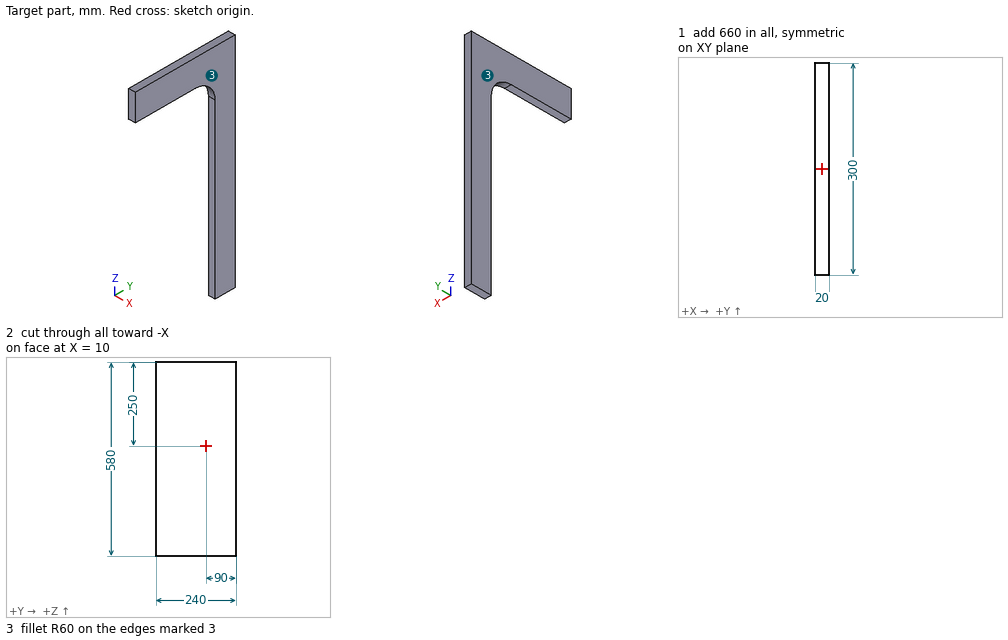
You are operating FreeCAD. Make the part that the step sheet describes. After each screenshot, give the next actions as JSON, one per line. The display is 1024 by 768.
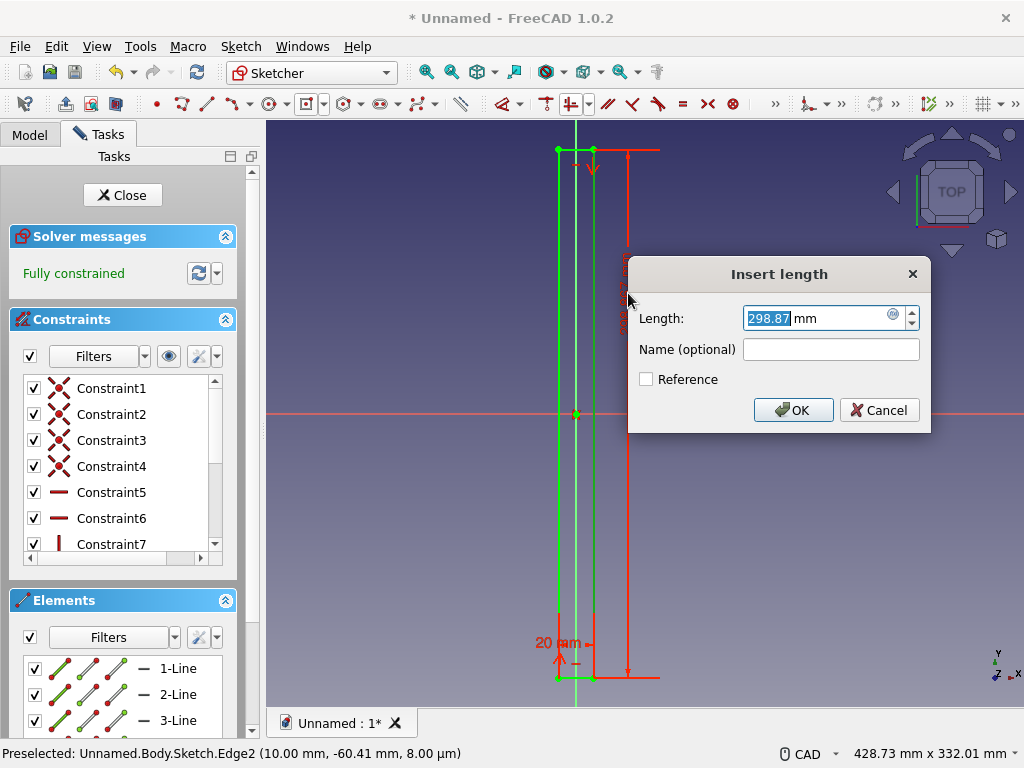
{"action": "type", "text": "300"}
{"action": "key", "text": "Return"}
{"action": "key", "text": "Escape"}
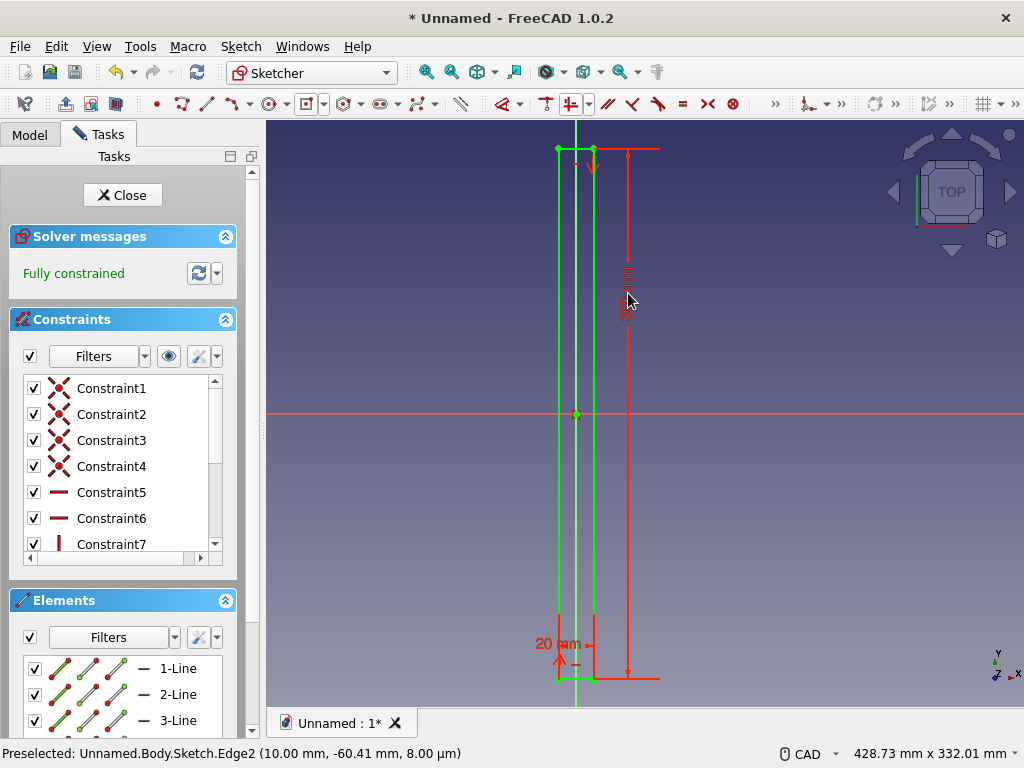
{"action": "left_click", "coordinate": [123, 195]}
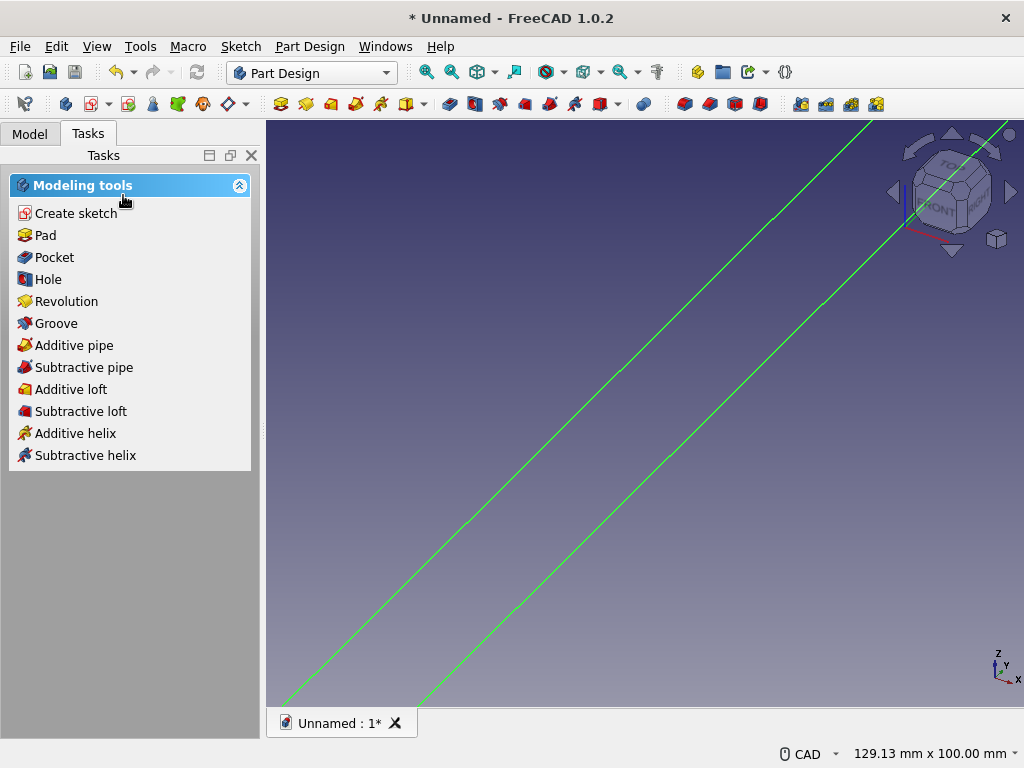
{"action": "left_click", "coordinate": [281, 104]}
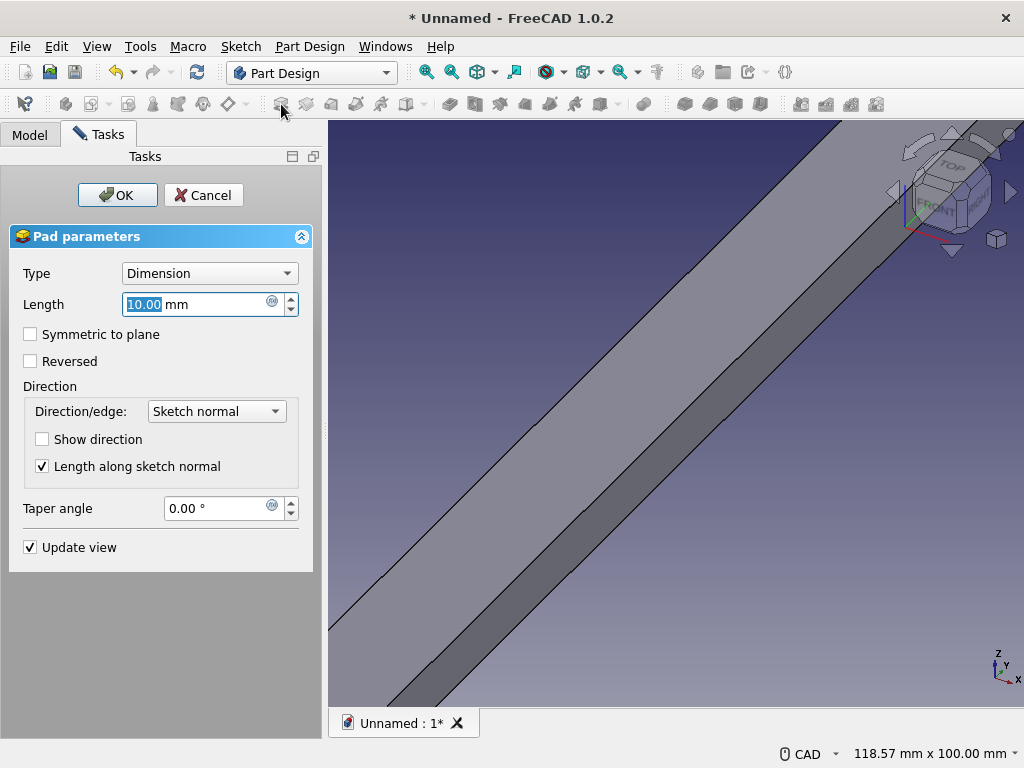
{"action": "type", "text": "660"}
{"action": "key", "text": "Tab"}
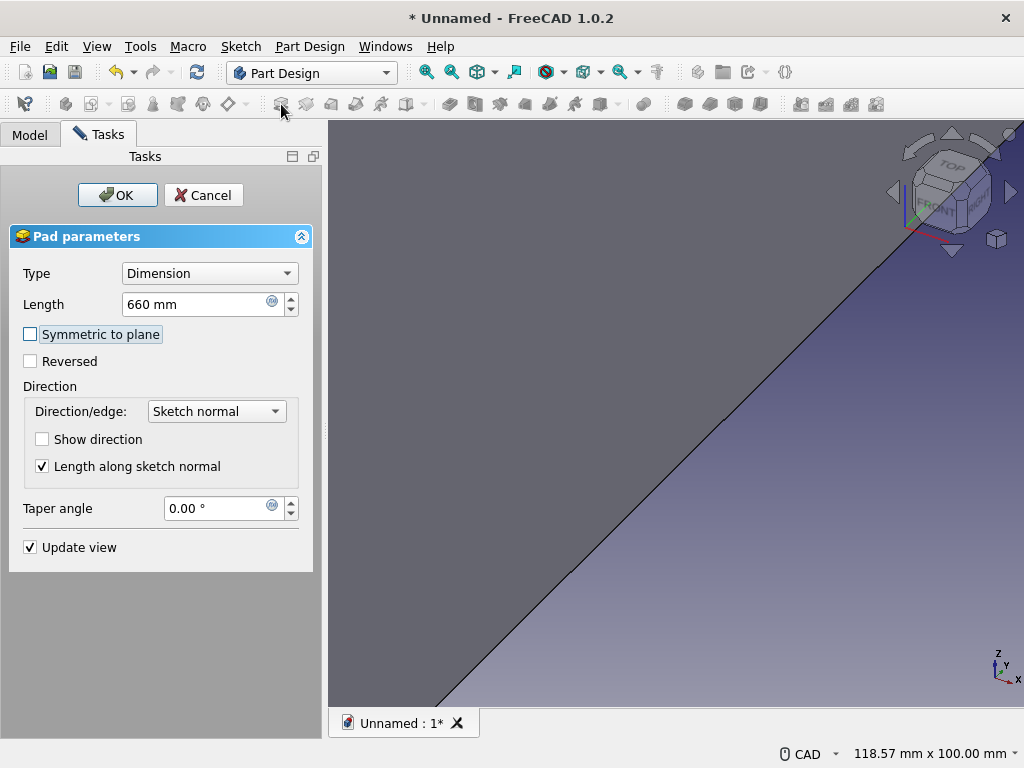
{"action": "left_click", "coordinate": [31, 334]}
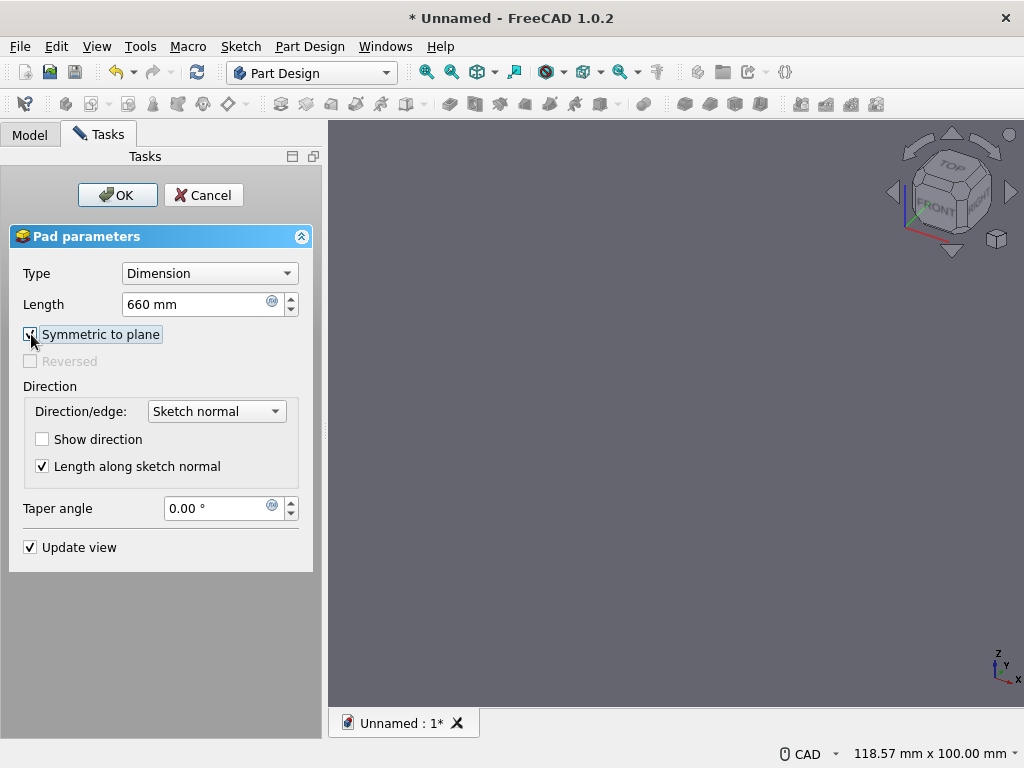
{"action": "left_click", "coordinate": [118, 195]}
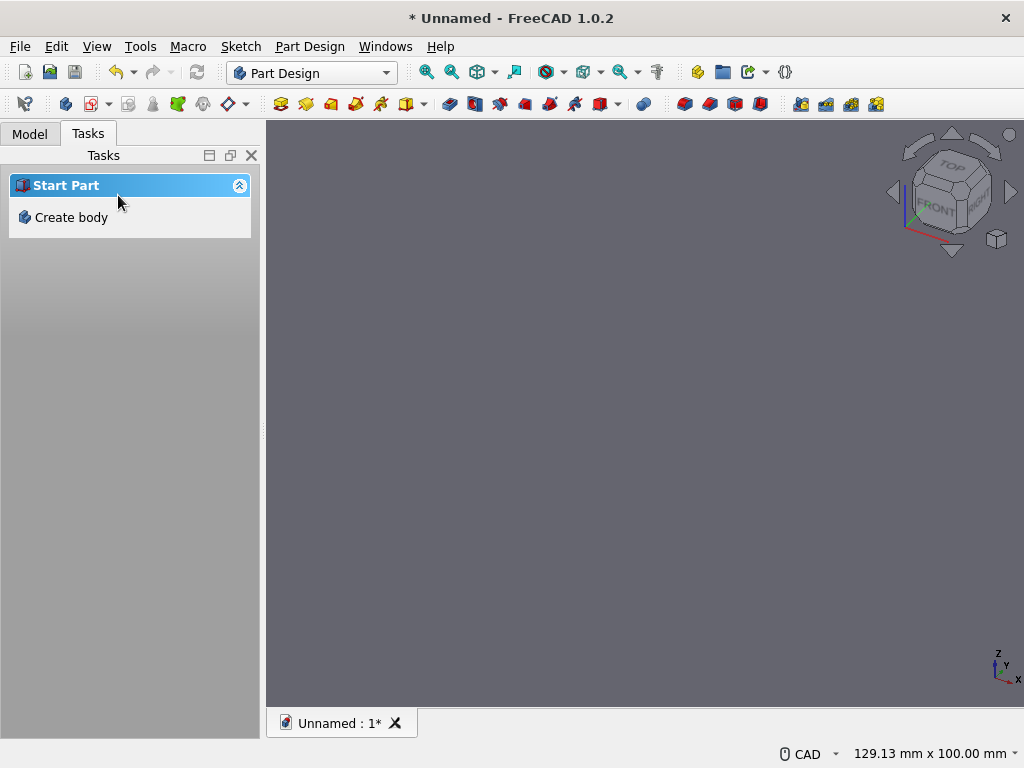
{"action": "left_click", "coordinate": [427, 72]}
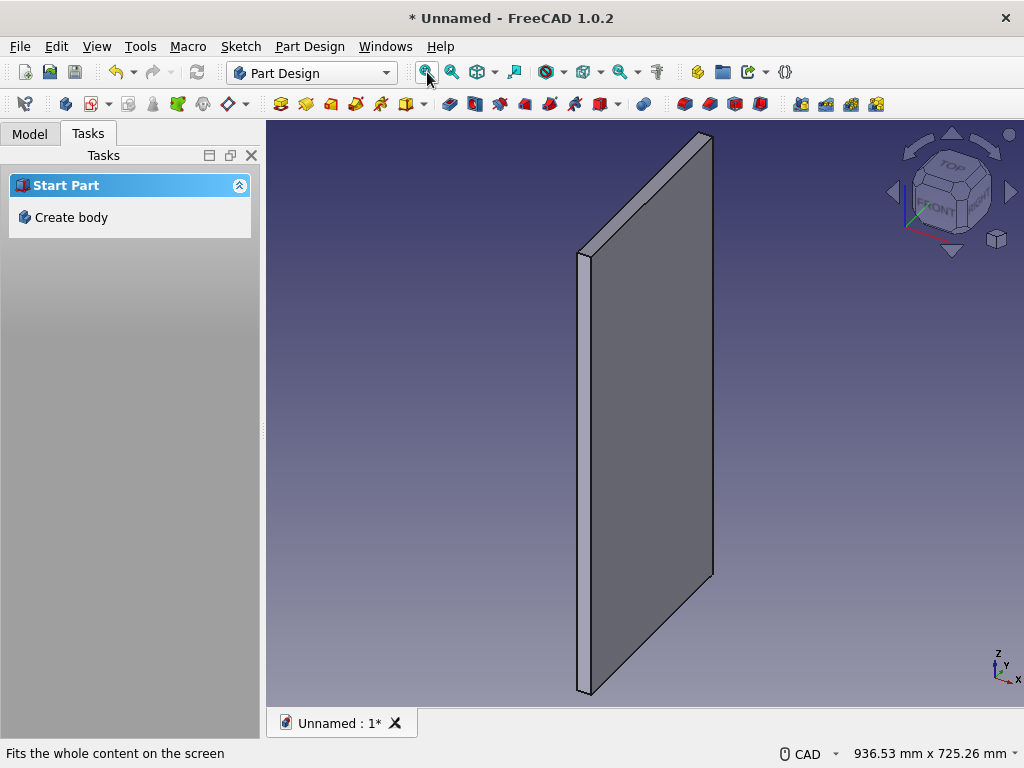
{"action": "left_click", "coordinate": [652, 352]}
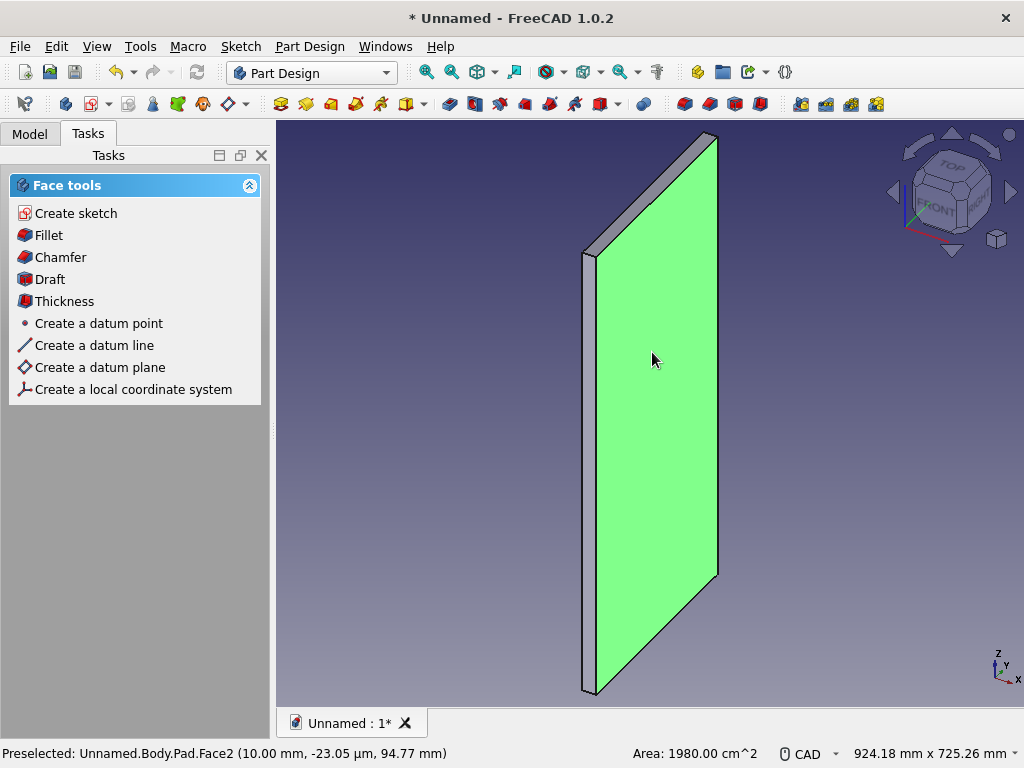
{"action": "left_click", "coordinate": [90, 104]}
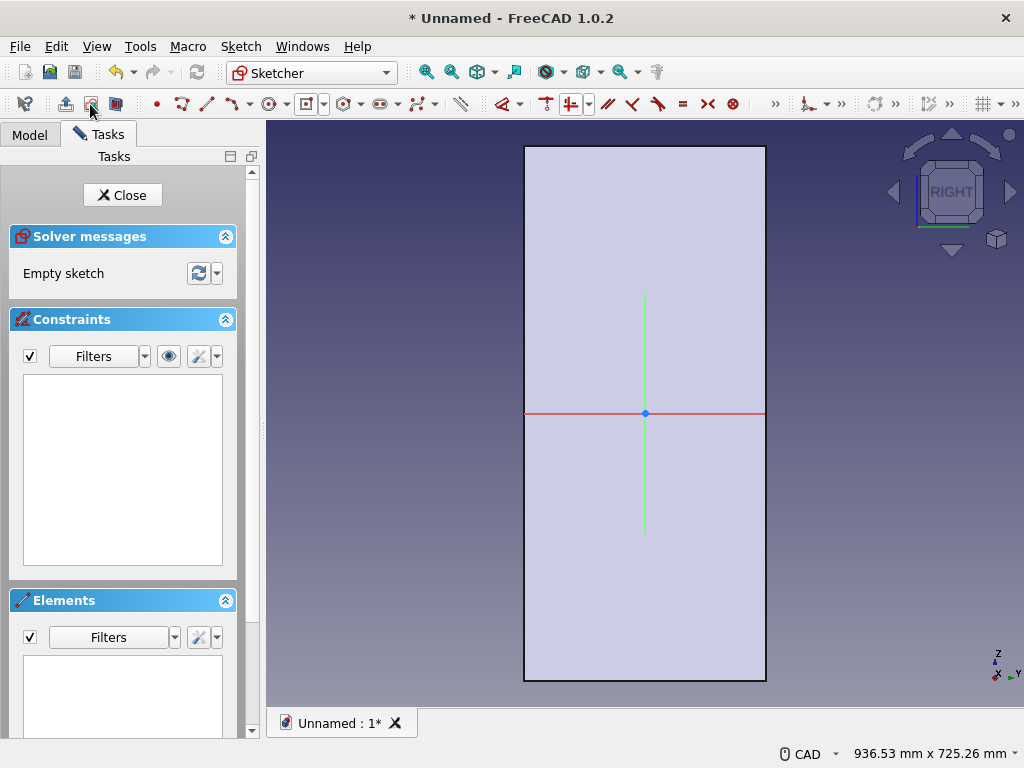
{"action": "scroll", "coordinate": [377, 267], "scroll_direction": "down", "scroll_amount": 1}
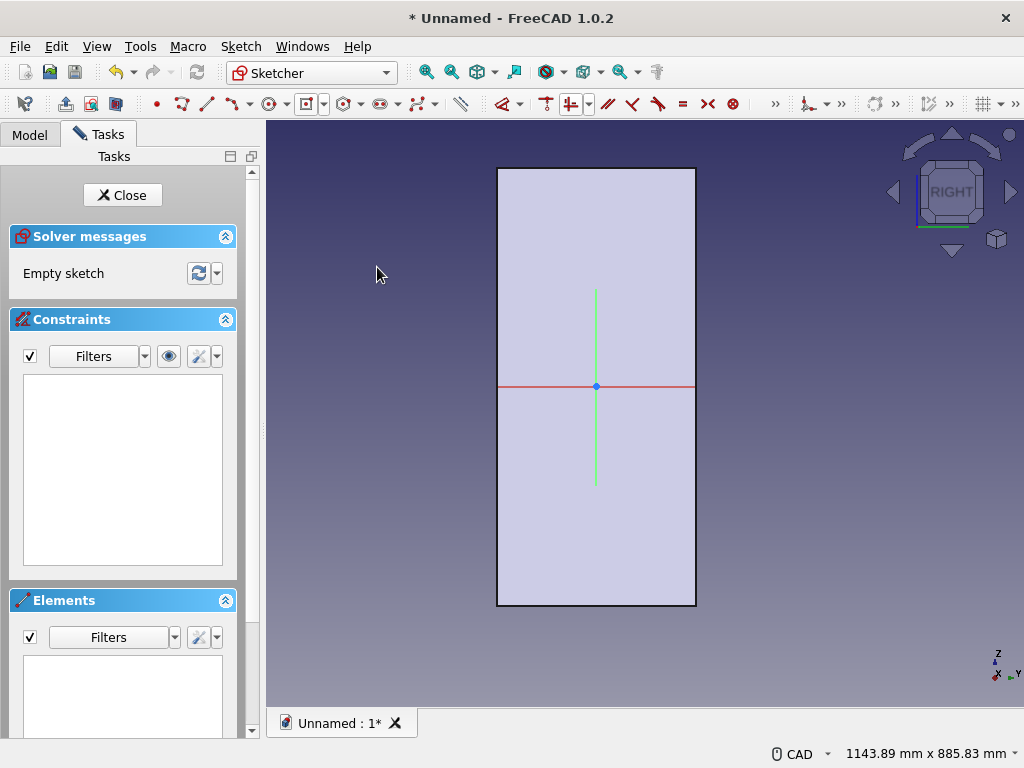
{"action": "left_click", "coordinate": [324, 104]}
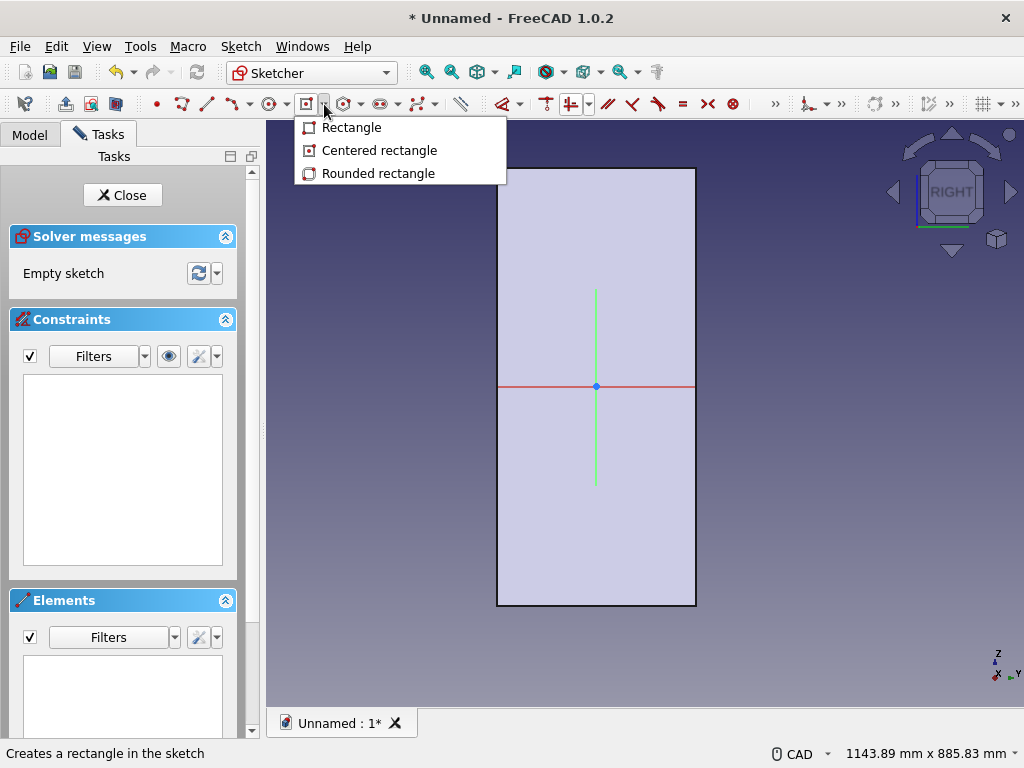
{"action": "left_click", "coordinate": [400, 128]}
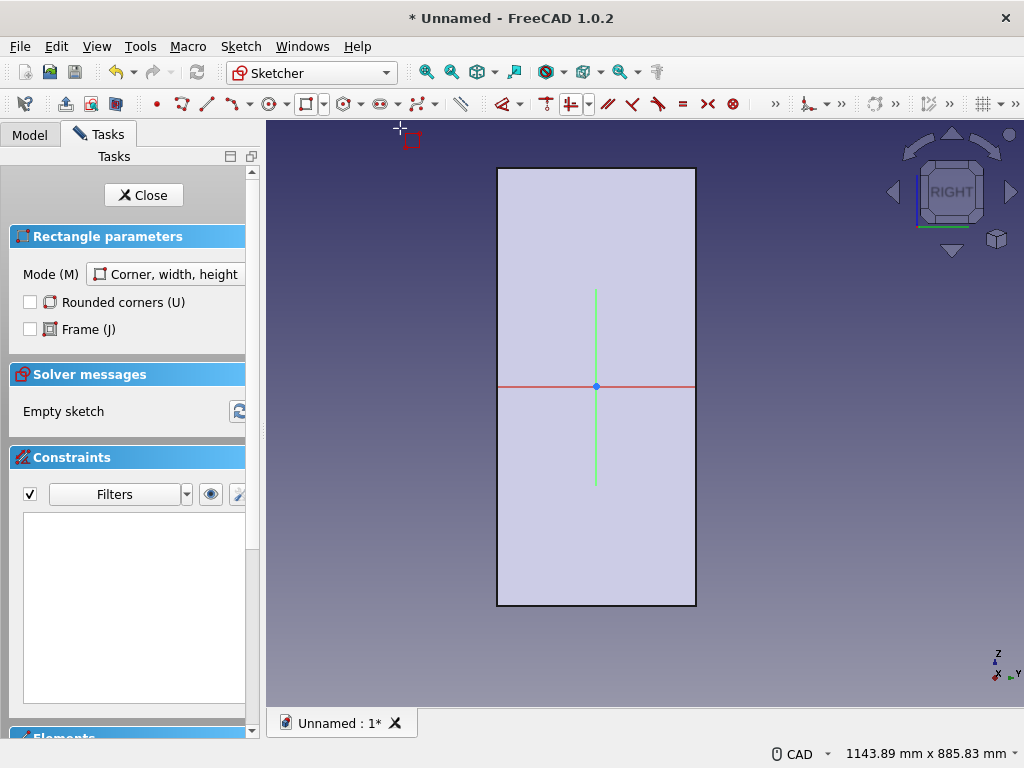
{"action": "left_click", "coordinate": [497, 221]}
{"action": "left_click", "coordinate": [656, 606]}
{"action": "key", "text": "Escape"}